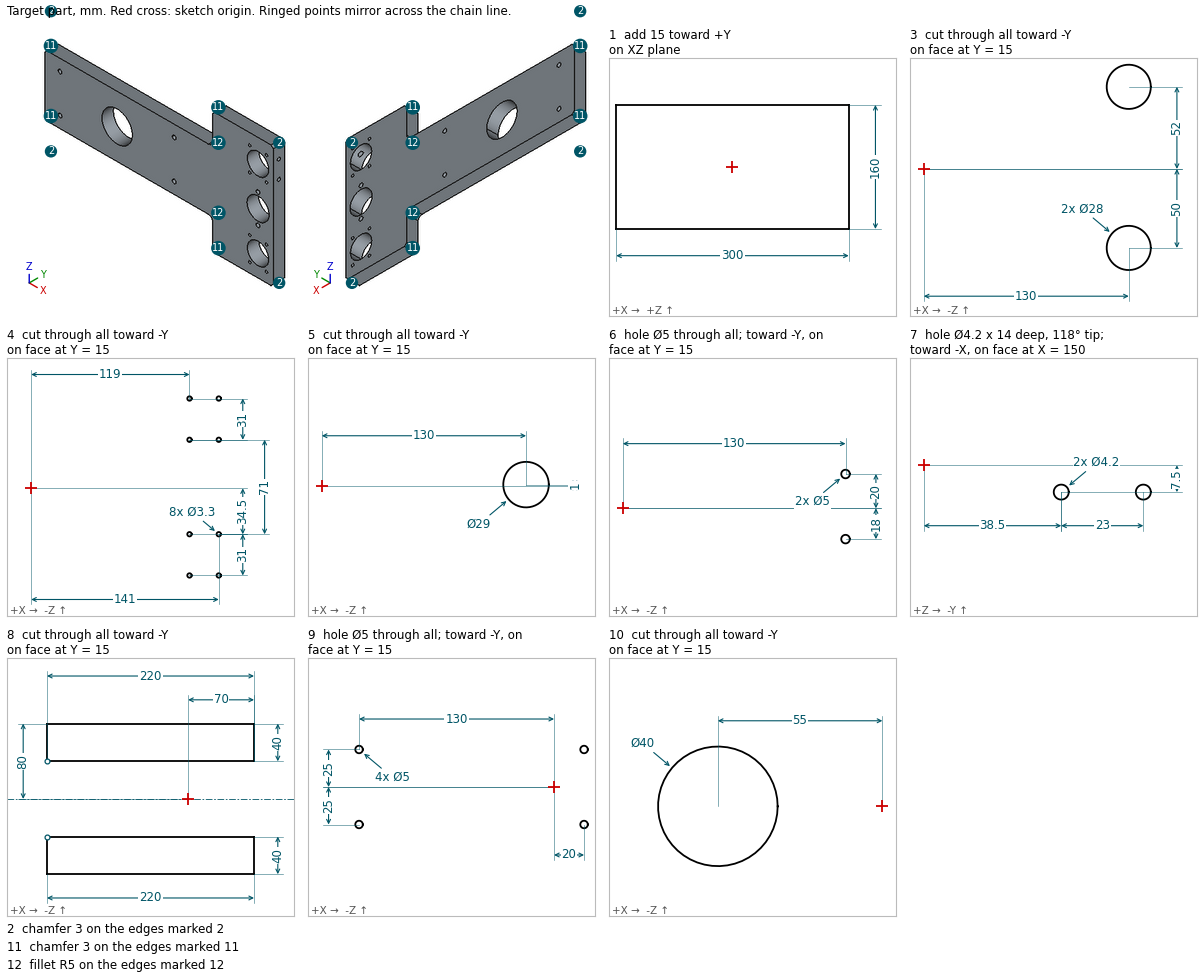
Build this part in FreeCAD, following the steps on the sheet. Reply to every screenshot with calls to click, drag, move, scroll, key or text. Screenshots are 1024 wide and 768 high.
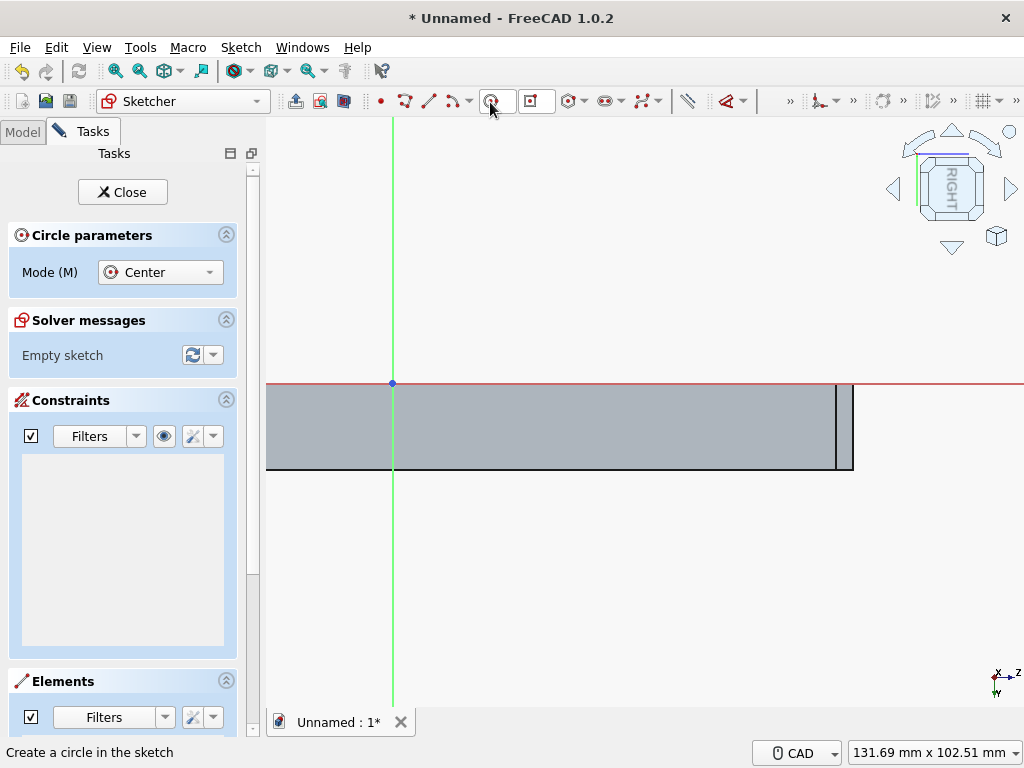
scroll(615, 427, up, 4)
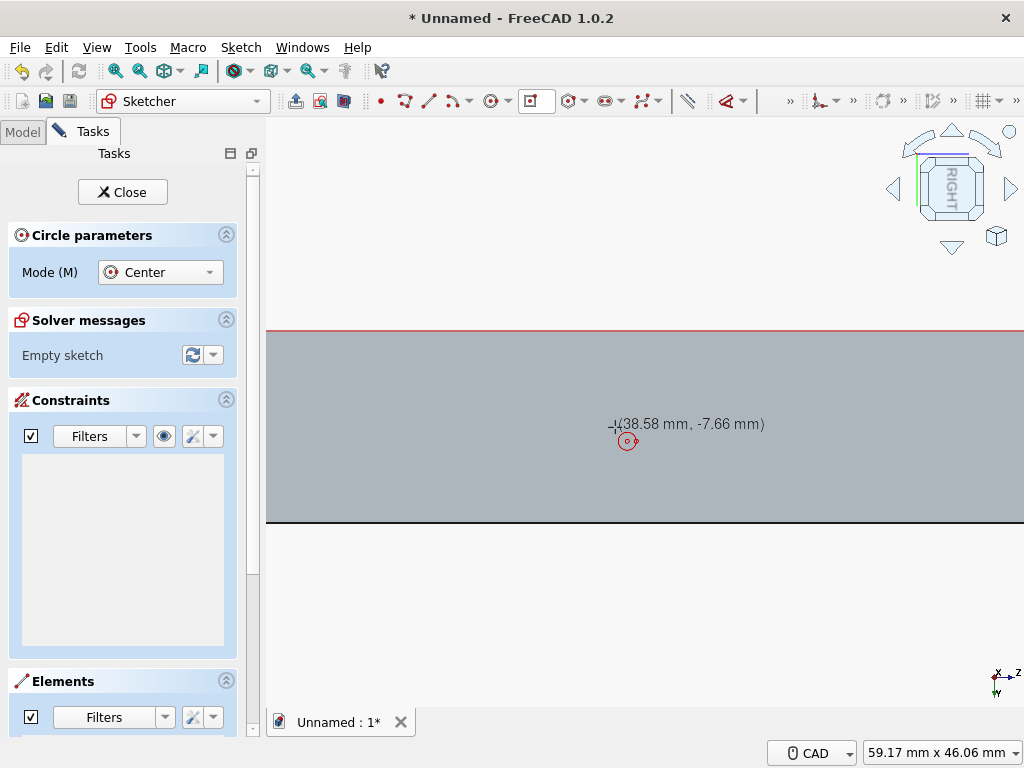
click(613, 427)
move(632, 408)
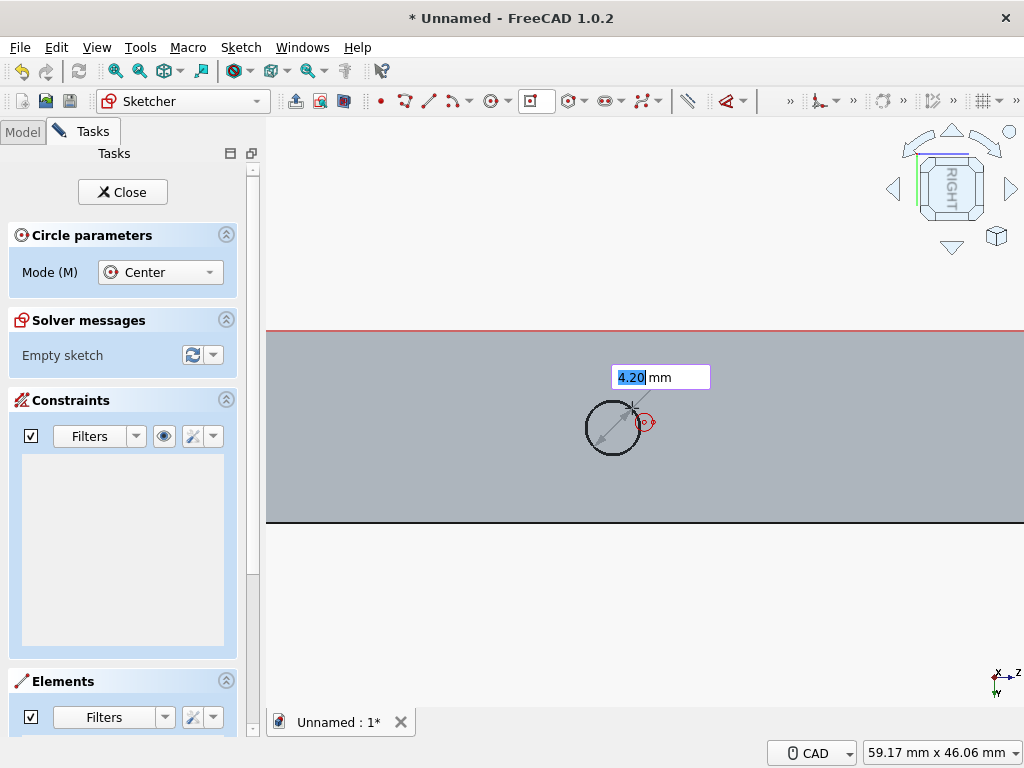
text(4.2)
key(Return)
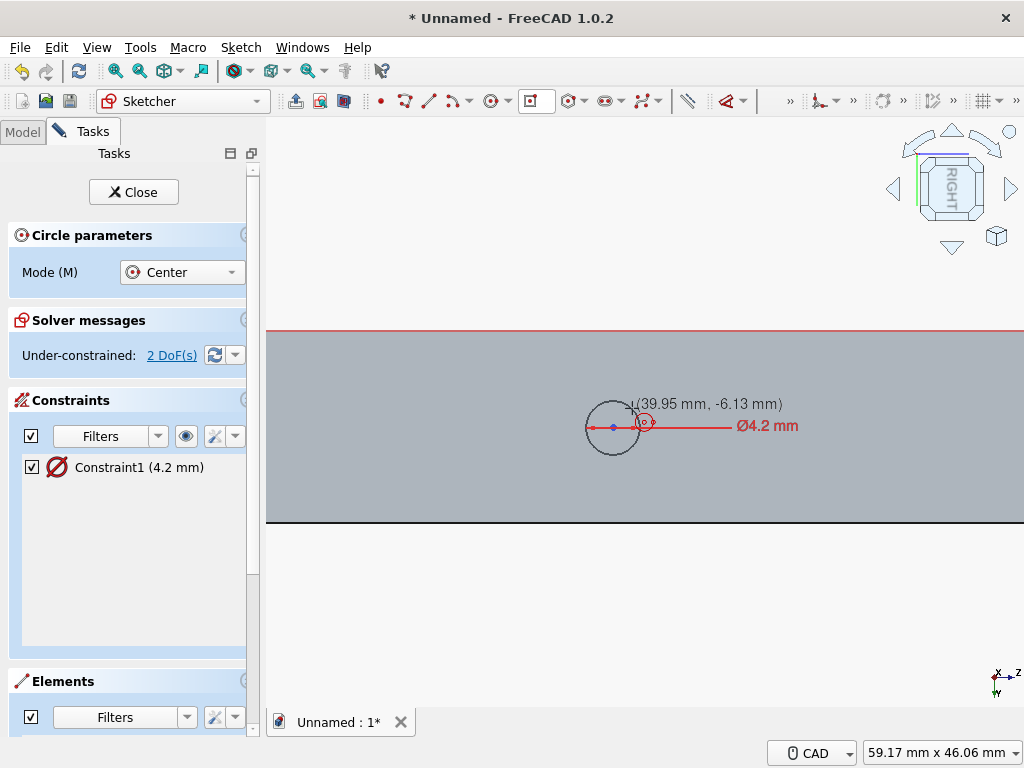
scroll(616, 428, down, 4)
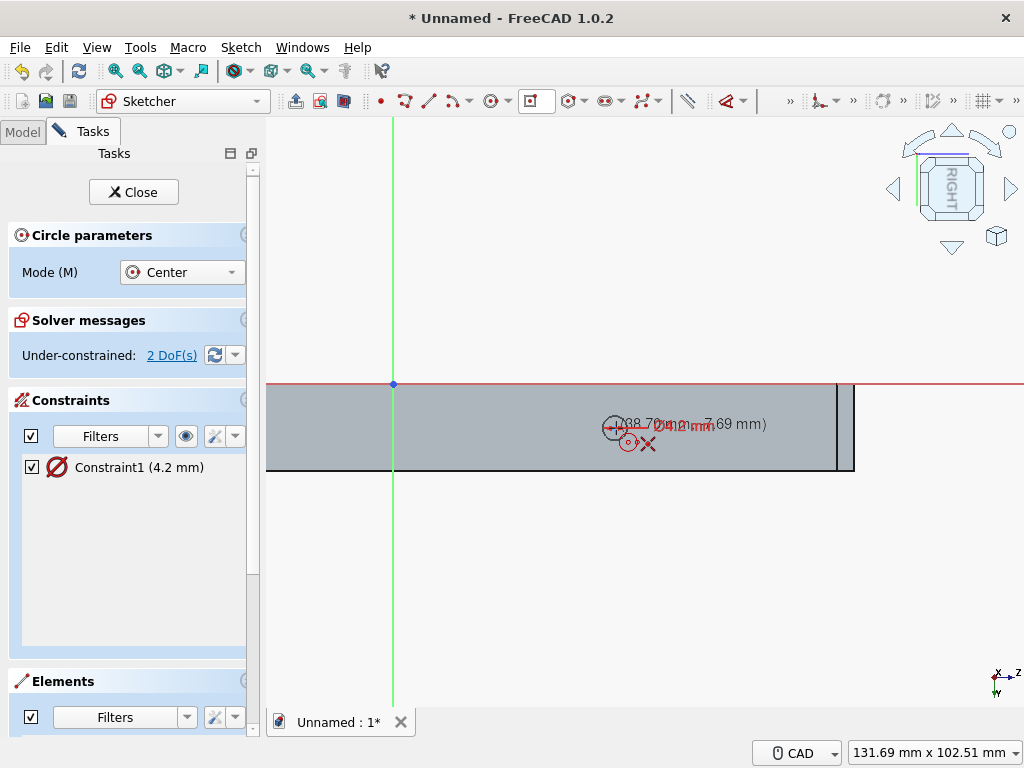
scroll(747, 428, up, 4)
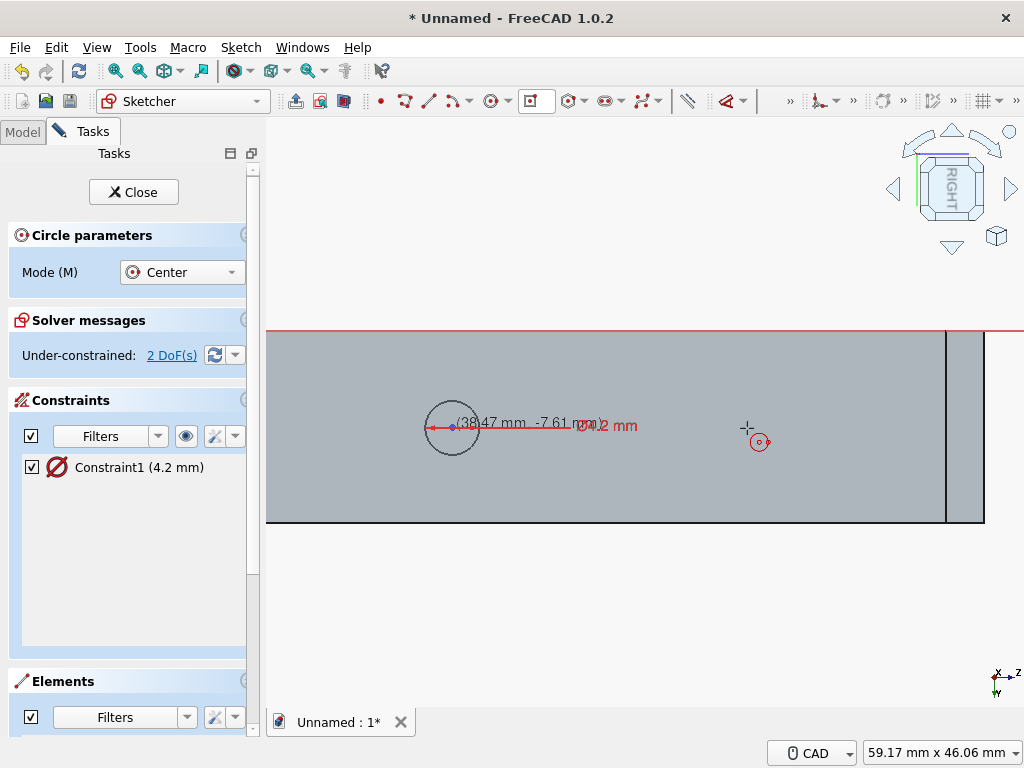
click(747, 427)
move(766, 408)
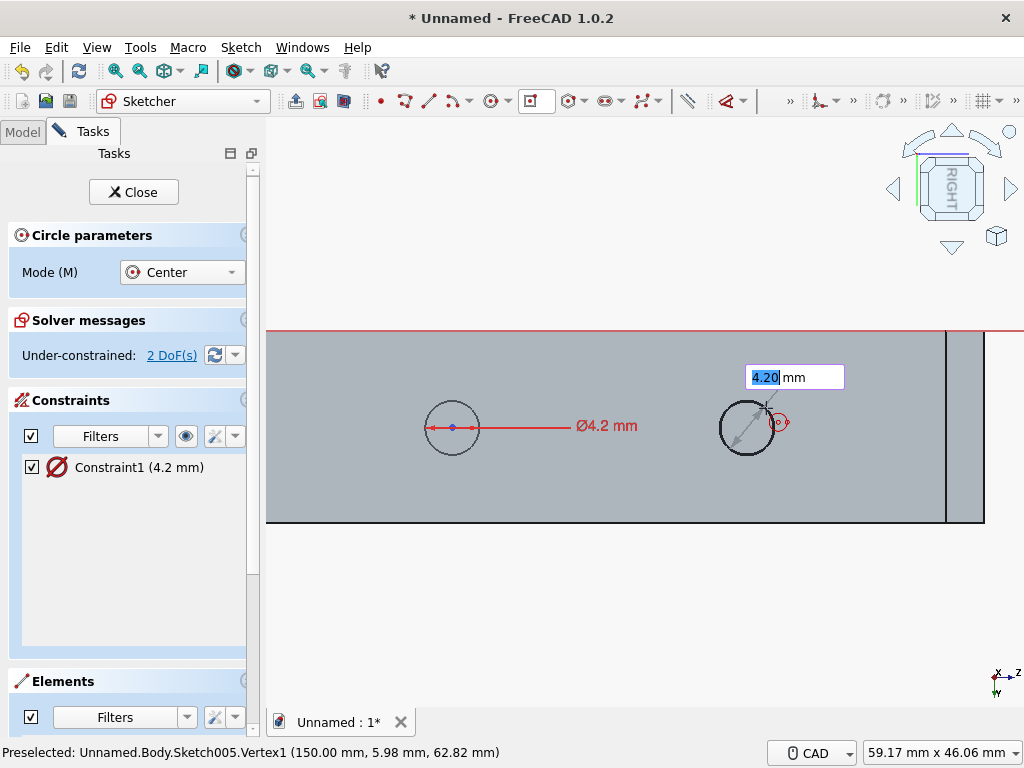
text(4.2)
key(Return)
key(Escape)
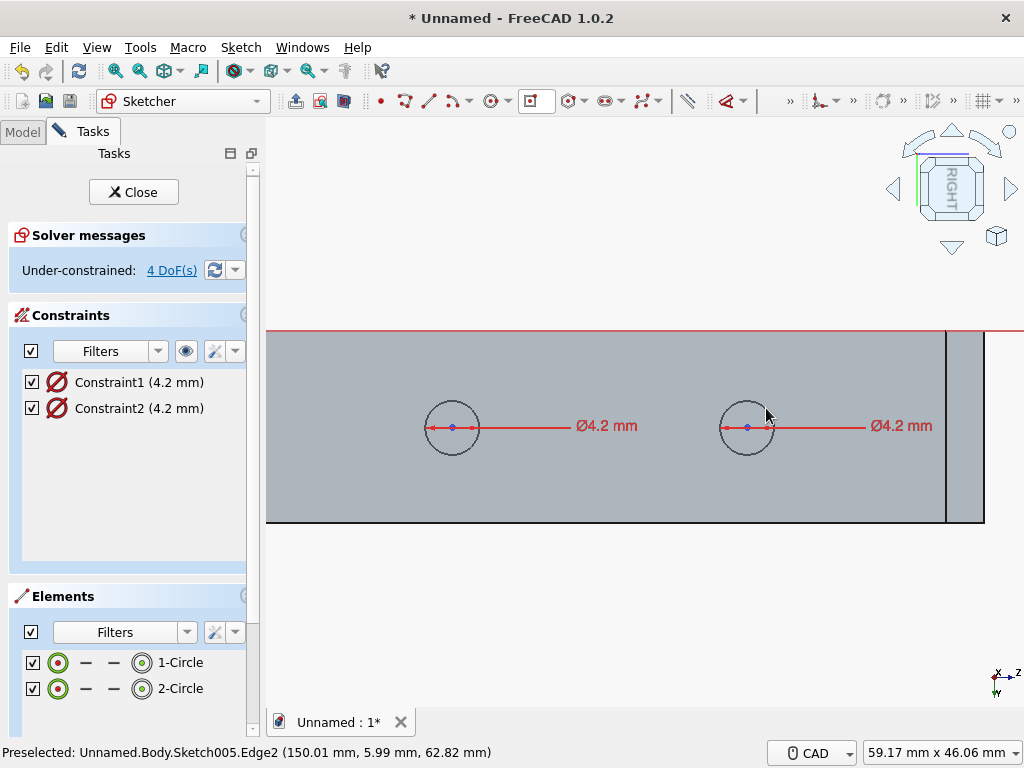
click(452, 428)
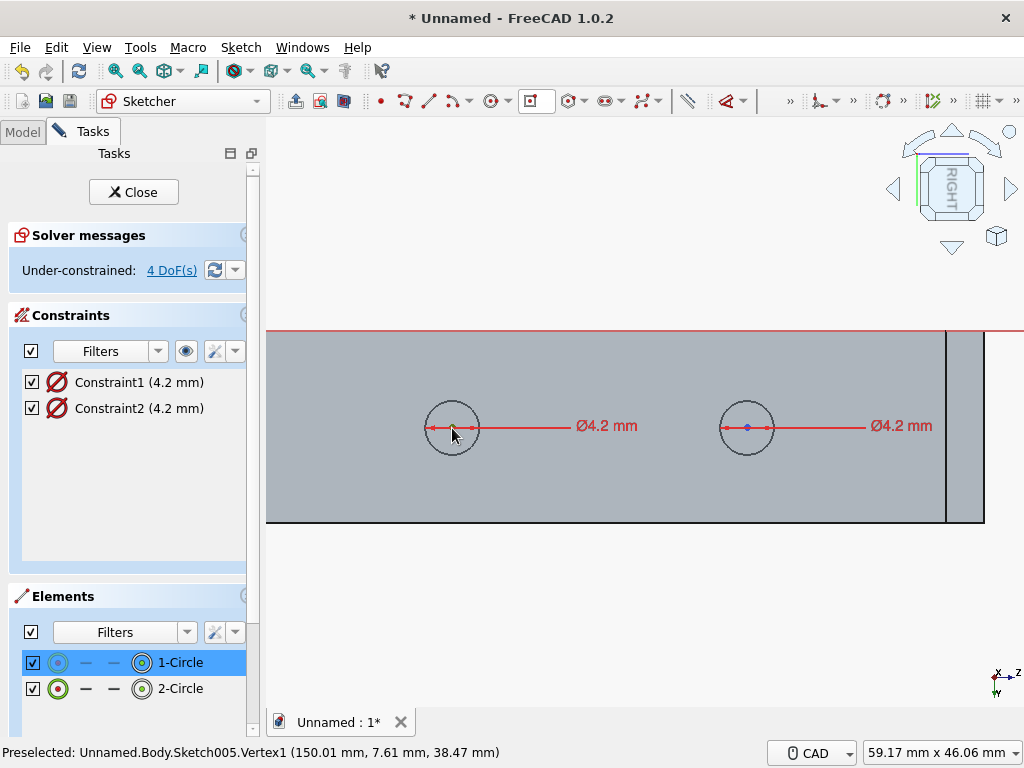
click(747, 428)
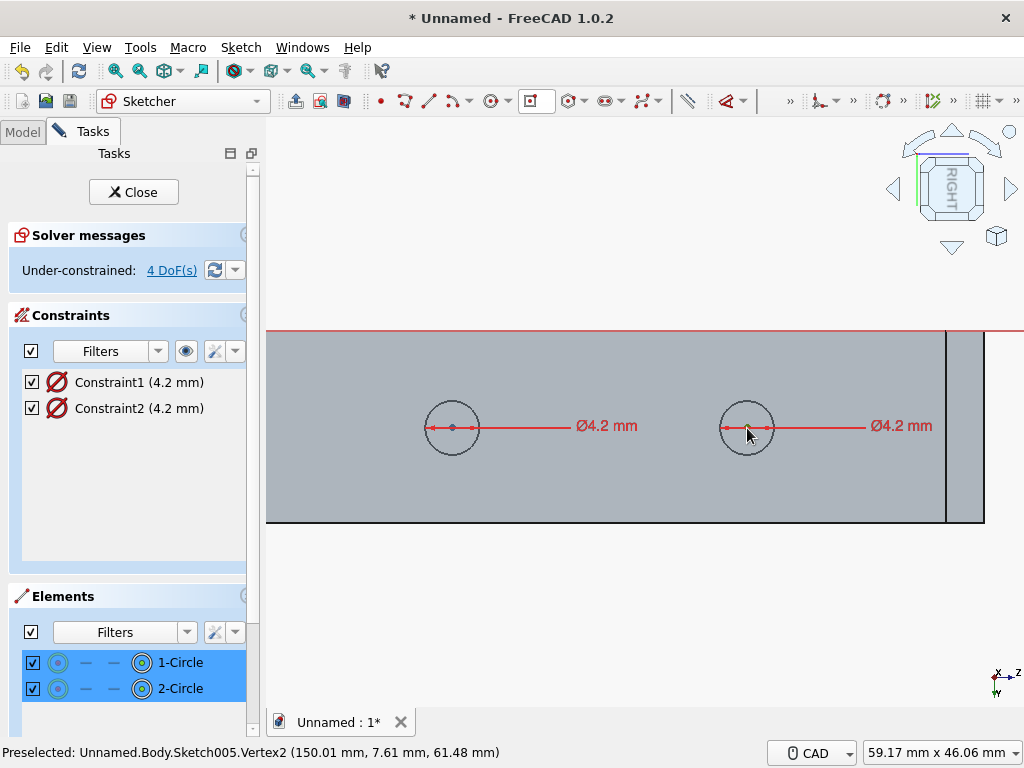
key(h)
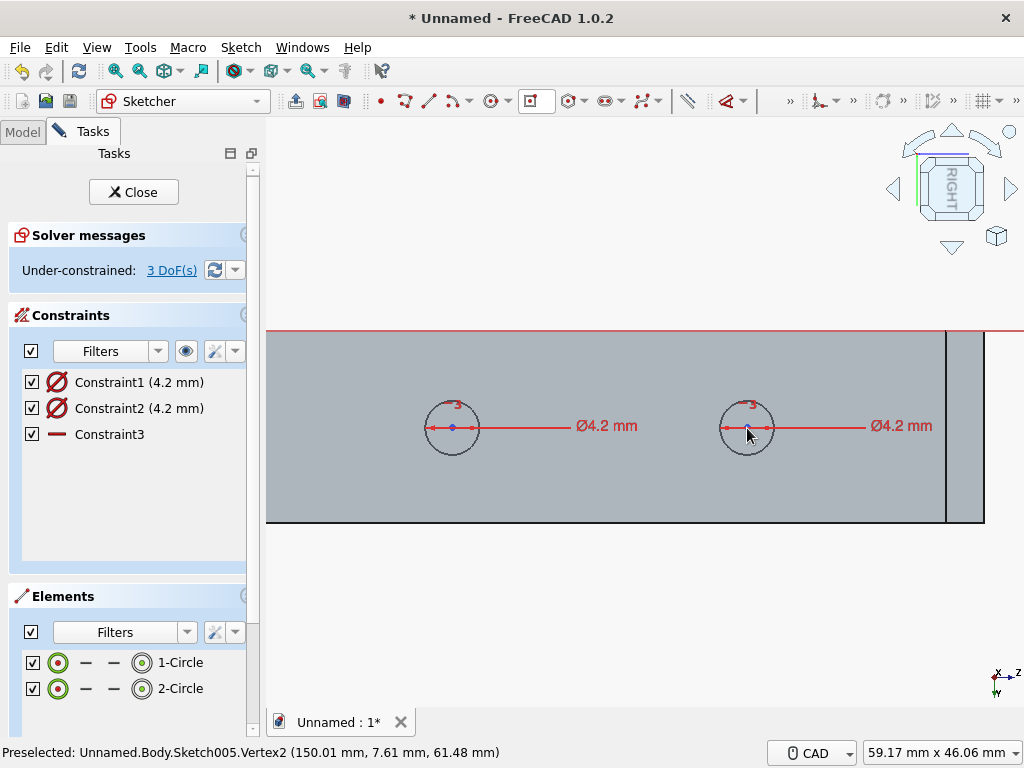
click(726, 102)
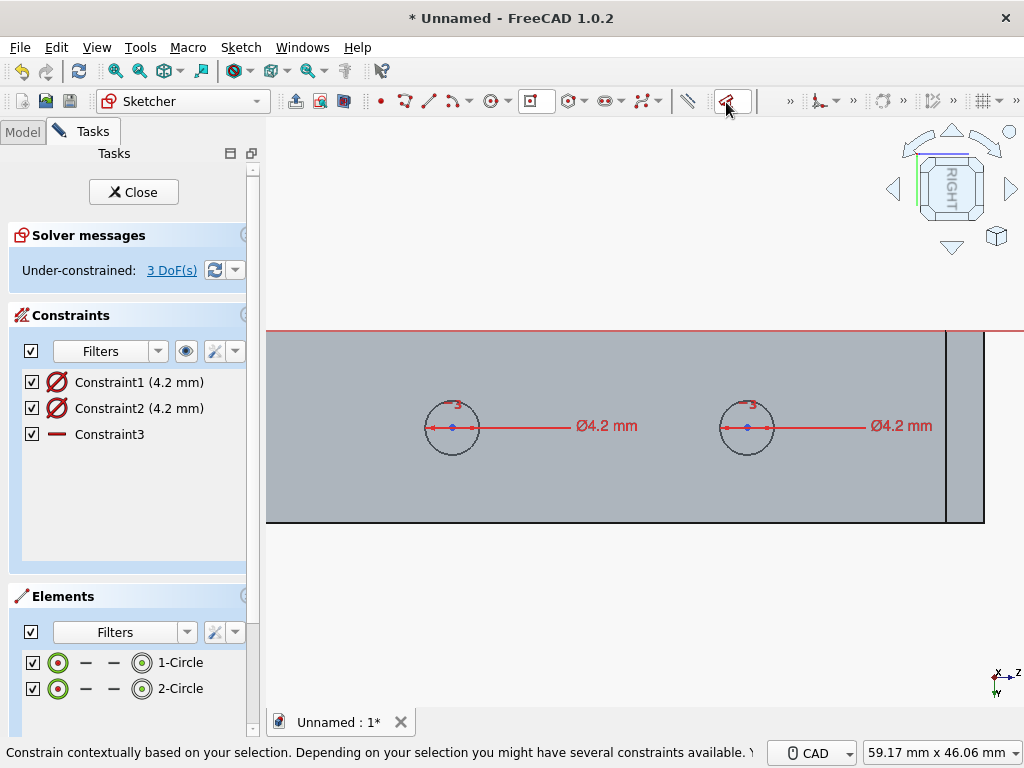
click(452, 428)
click(486, 379)